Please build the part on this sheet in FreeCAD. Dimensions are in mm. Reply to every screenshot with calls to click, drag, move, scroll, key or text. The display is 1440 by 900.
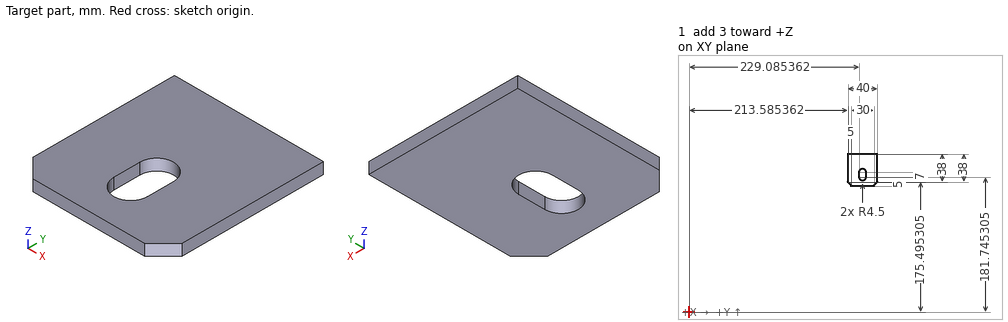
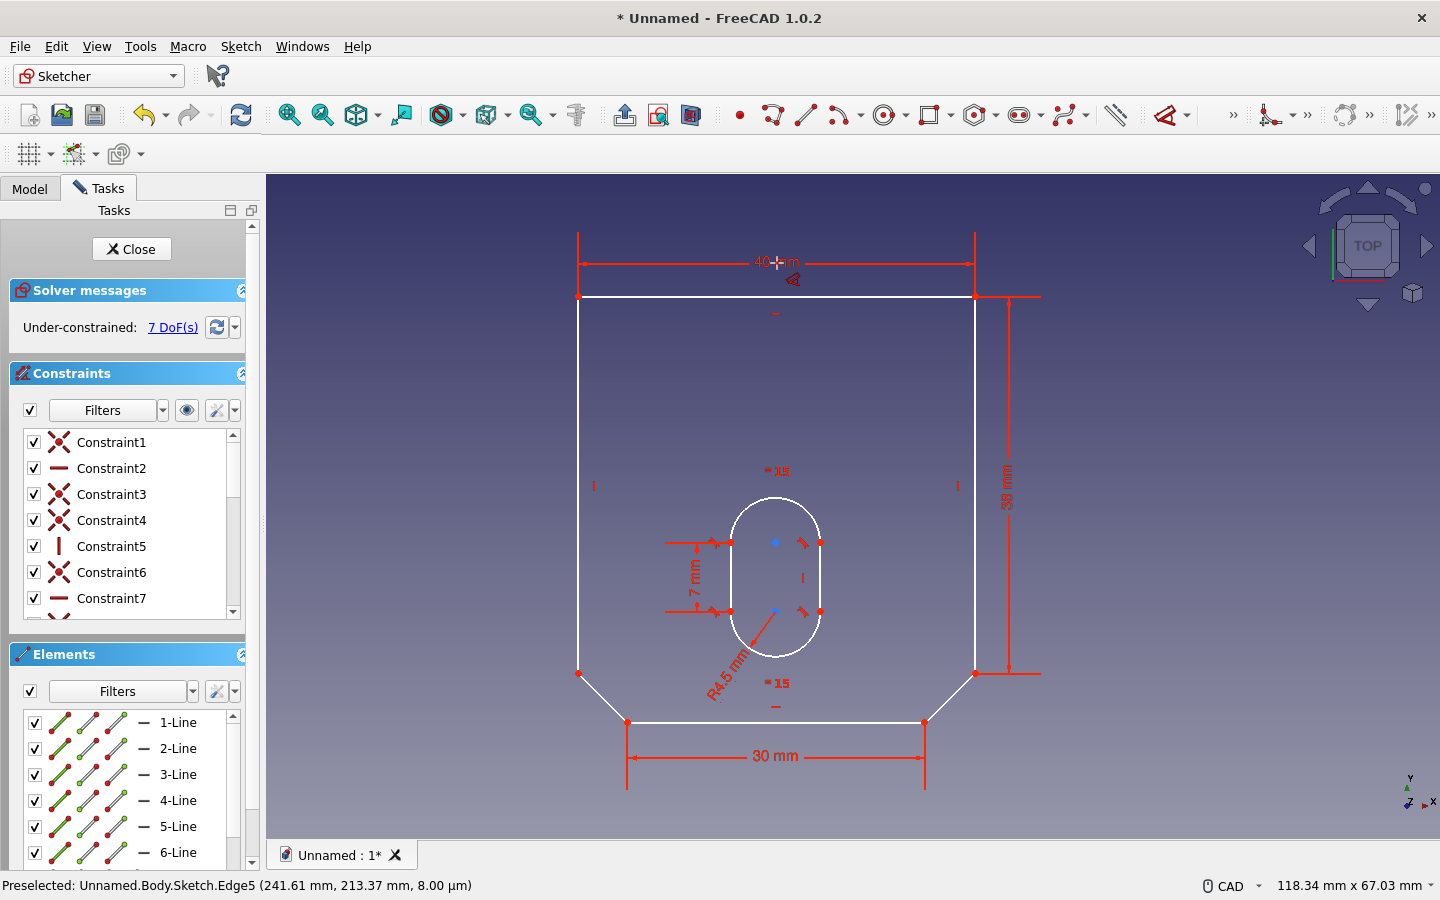
click(578, 410)
click(544, 486)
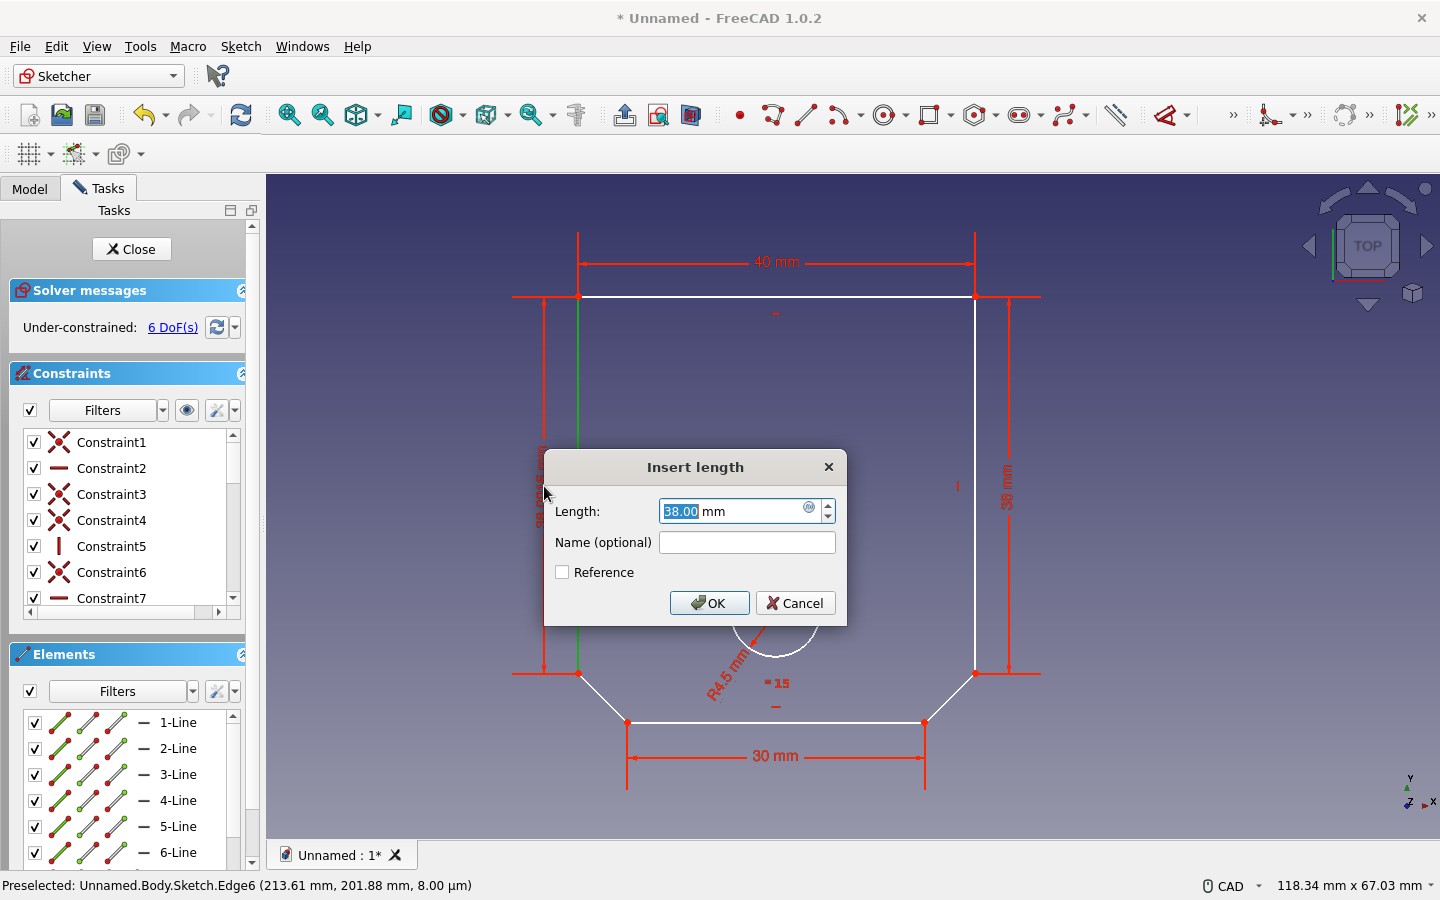
text(38)
key(Return)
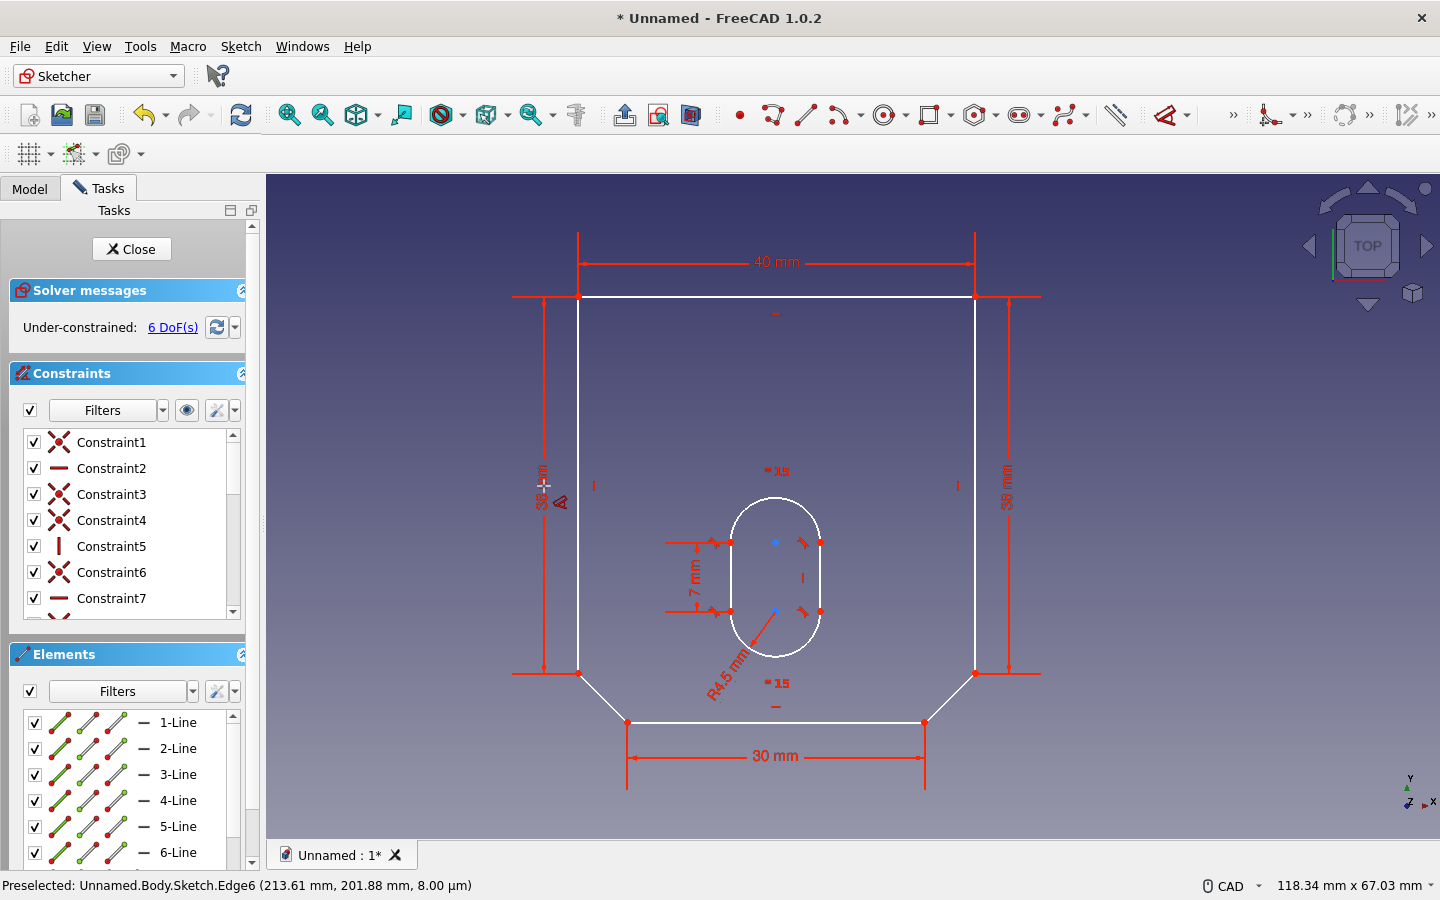
click(593, 689)
click(603, 757)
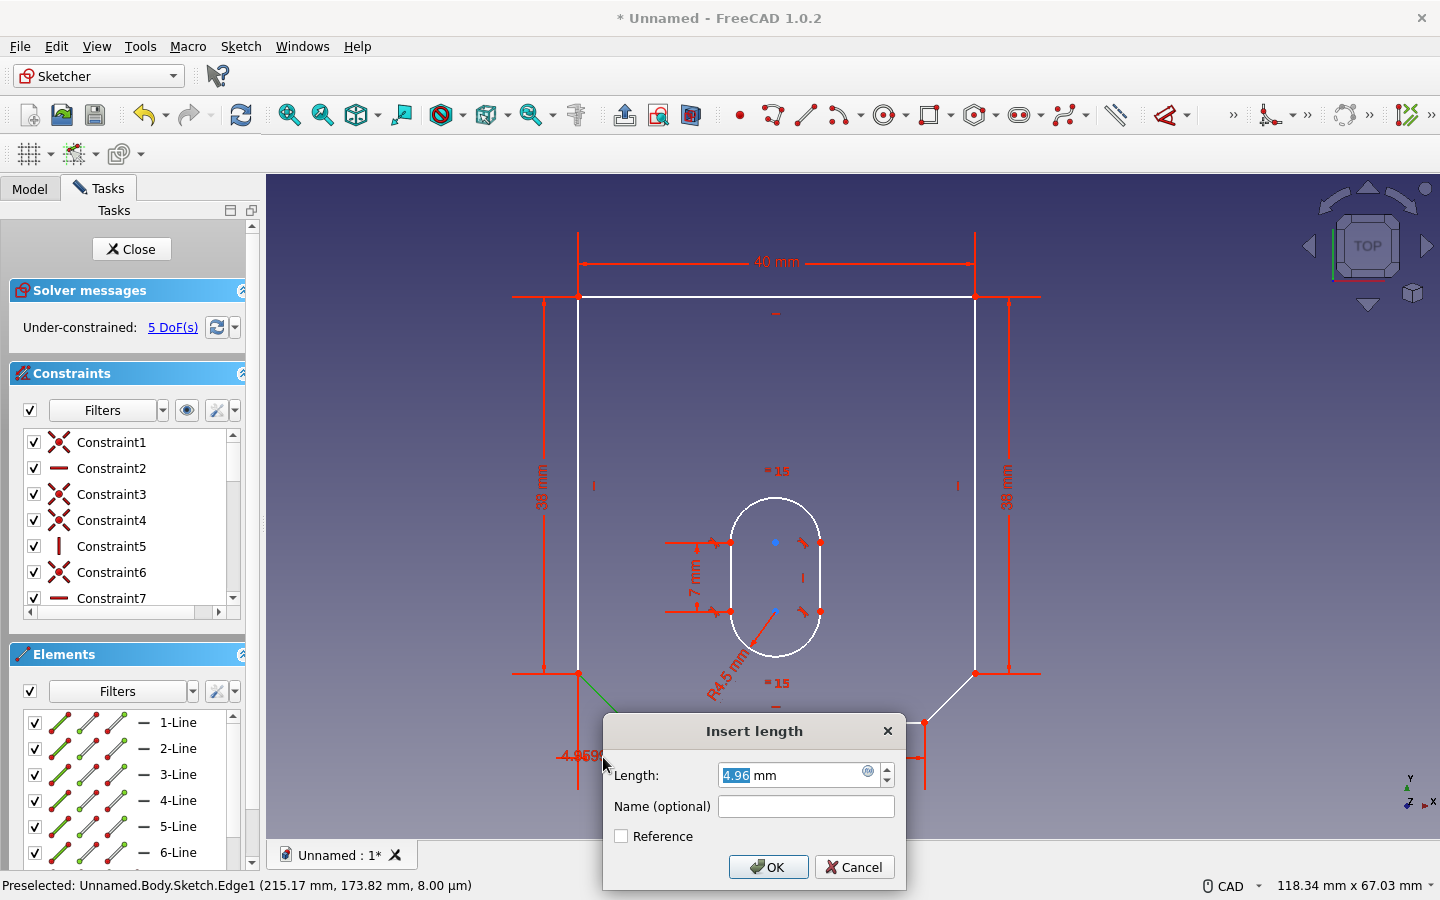
text(5)
key(Return)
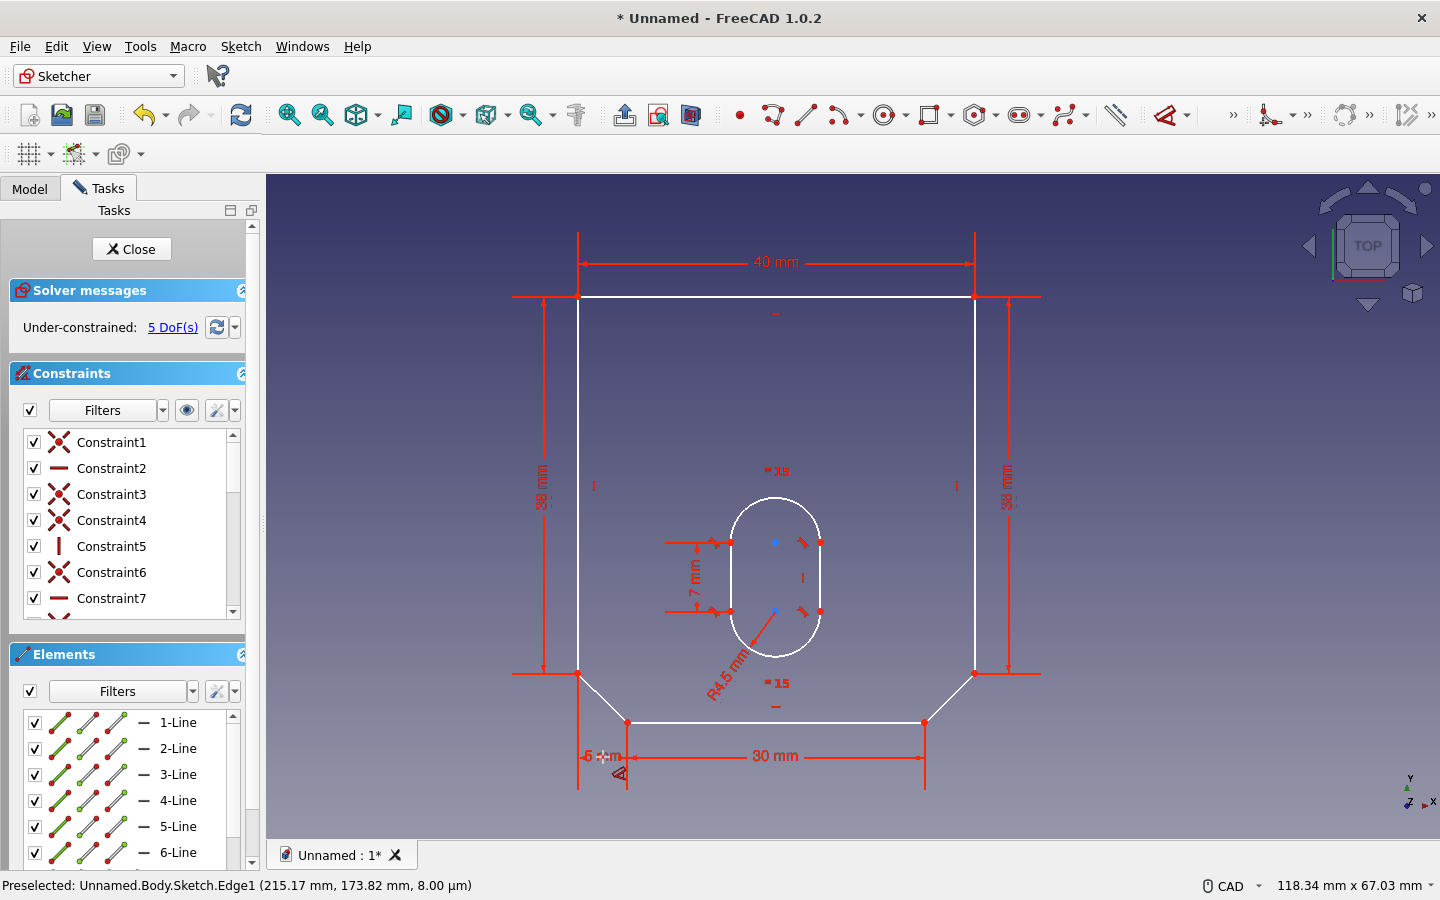
click(593, 689)
click(544, 698)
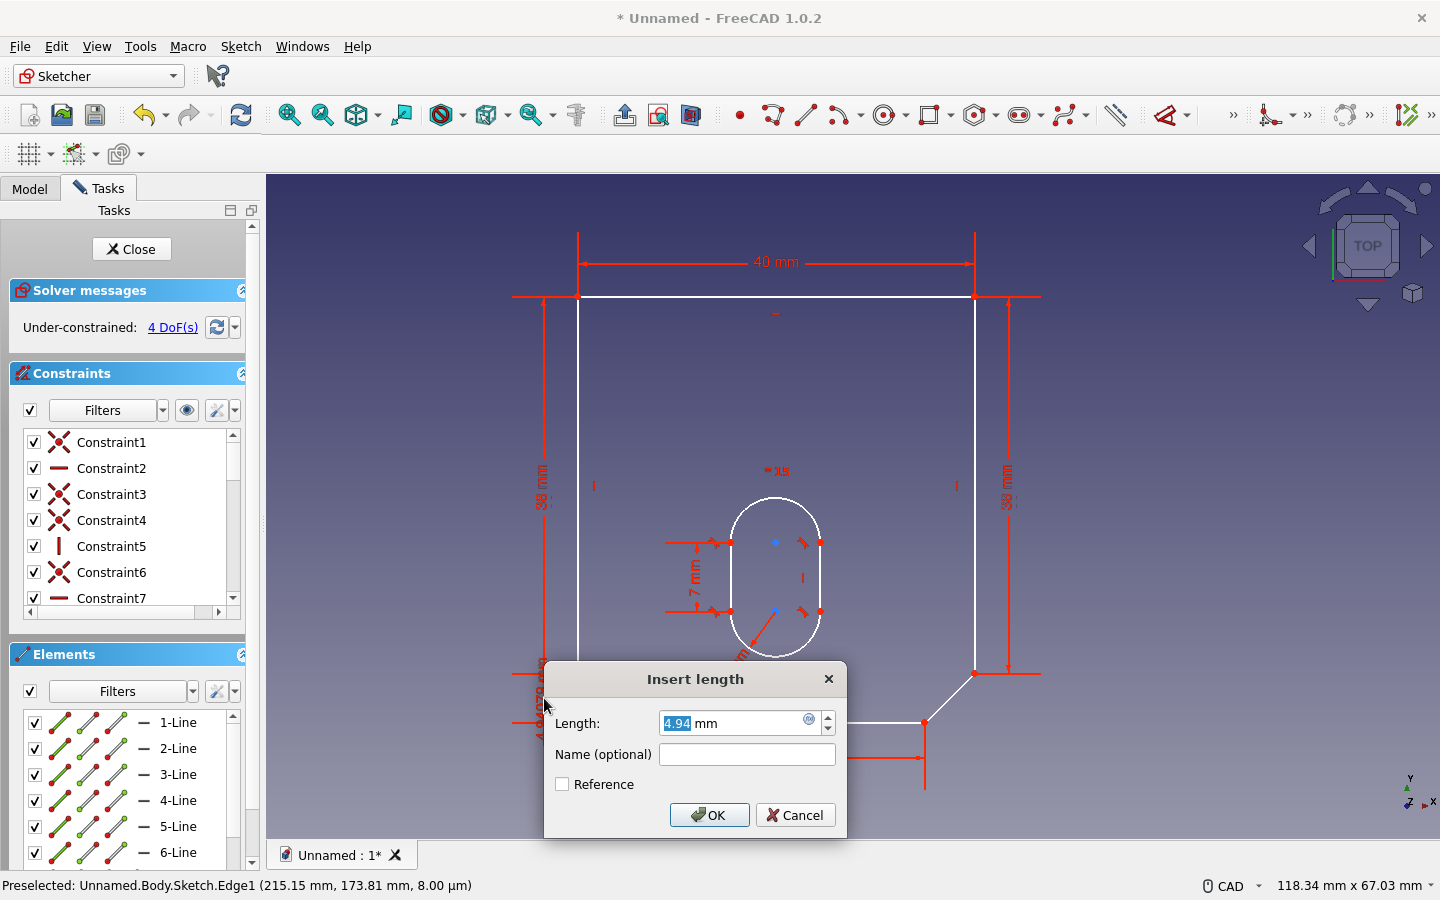
text(5)
key(Return)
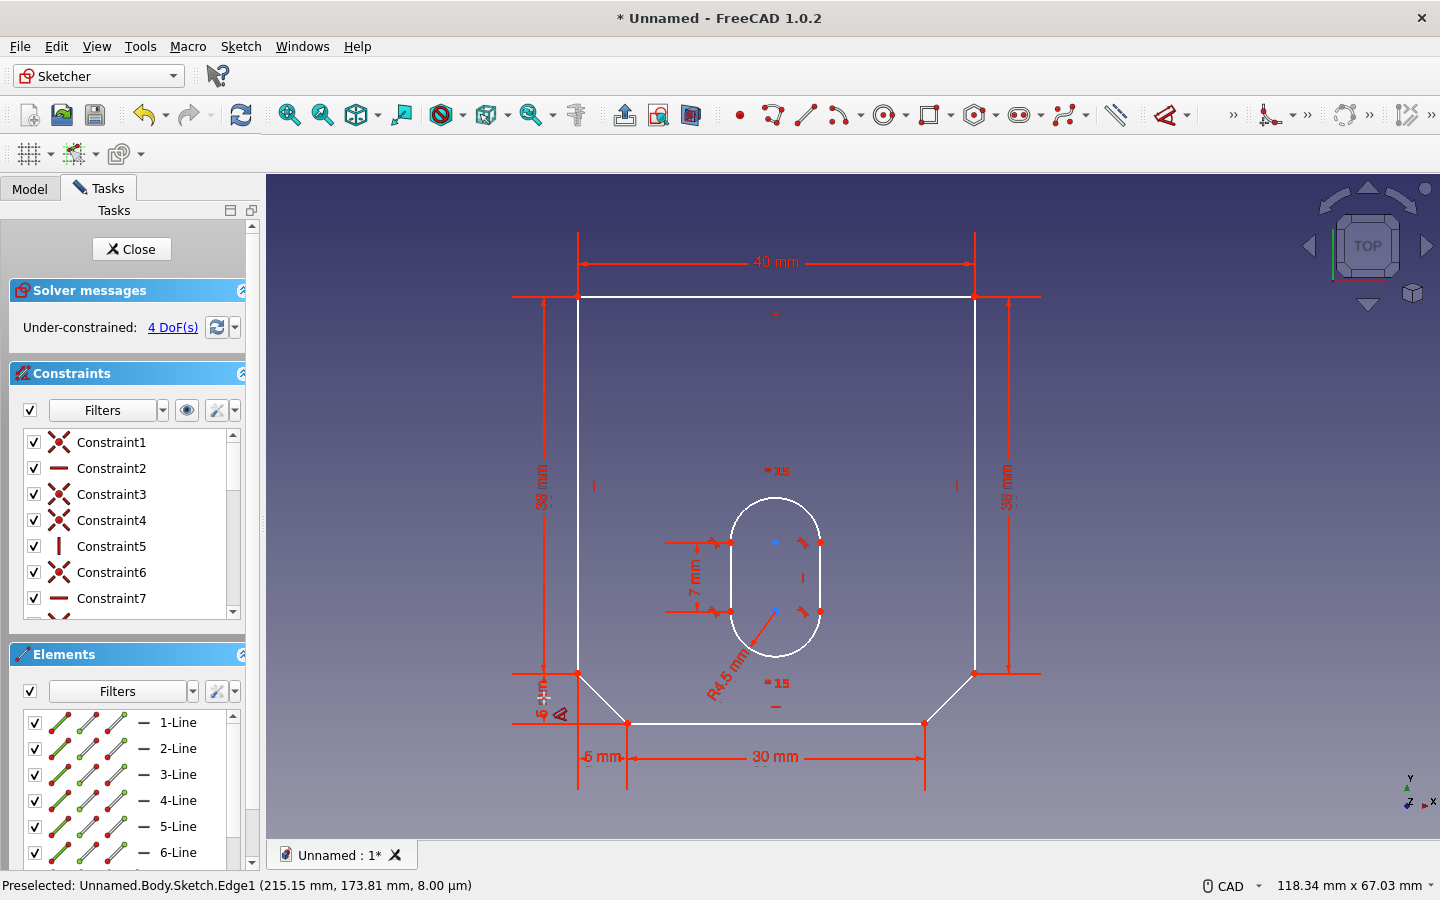
click(578, 674)
click(436, 640)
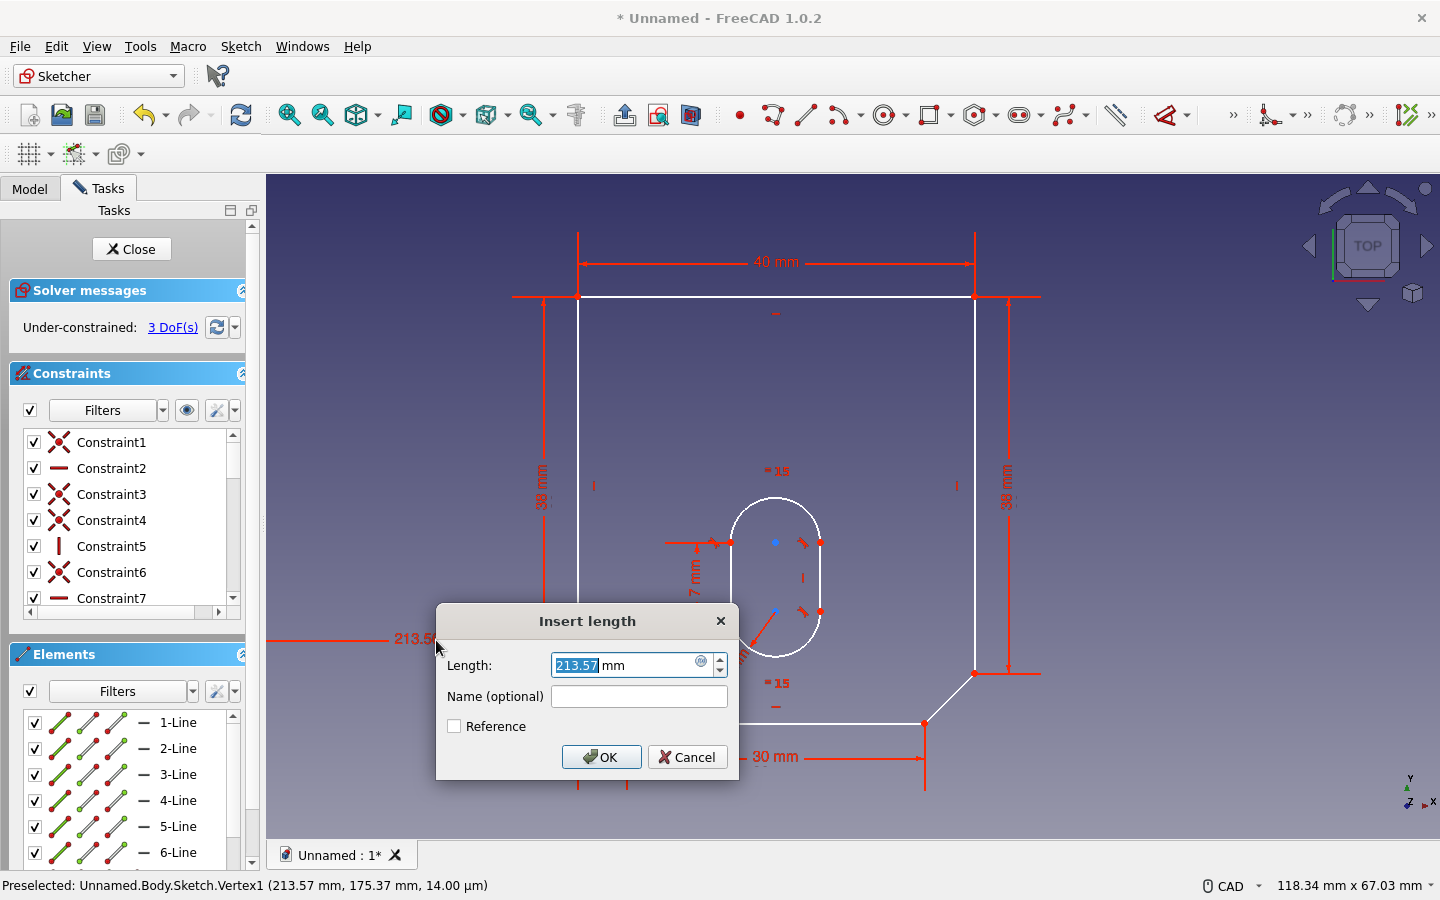
text(213.585362)
key(Return)